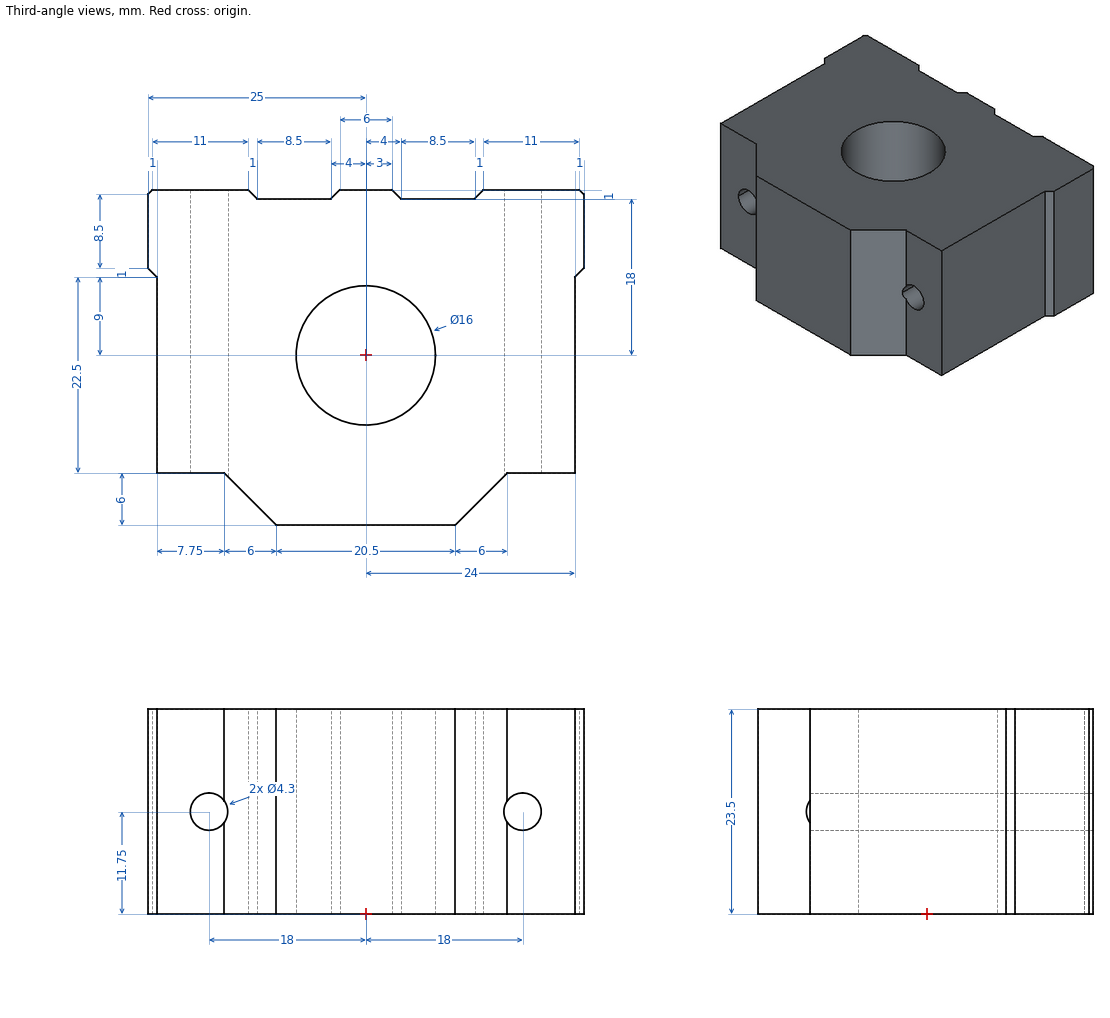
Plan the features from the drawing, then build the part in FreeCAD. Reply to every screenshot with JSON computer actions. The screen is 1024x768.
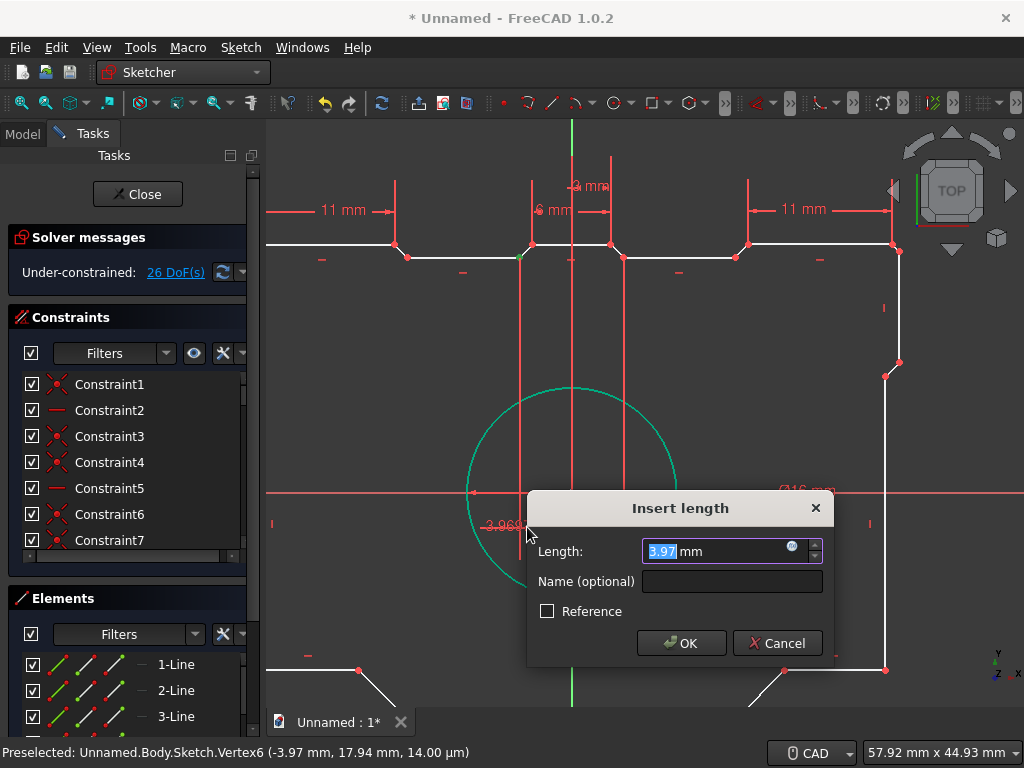
{"action": "type", "text": "4"}
{"action": "key", "text": "Return"}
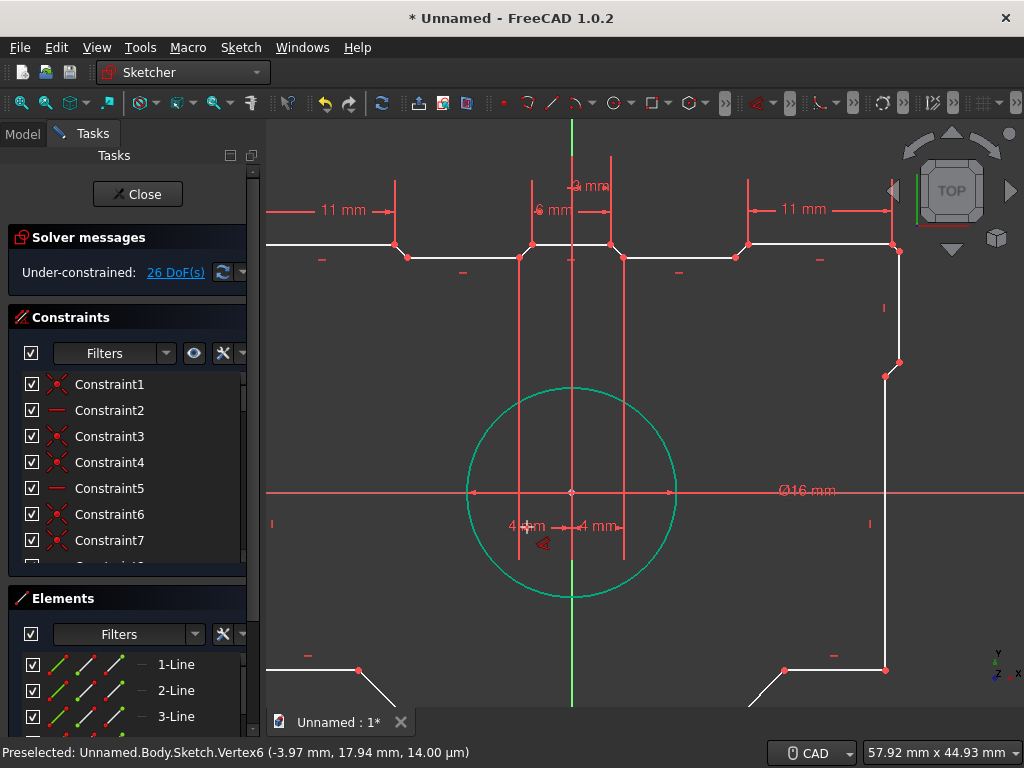
{"action": "scroll", "coordinate": [586, 244], "scroll_direction": "down", "scroll_amount": 2}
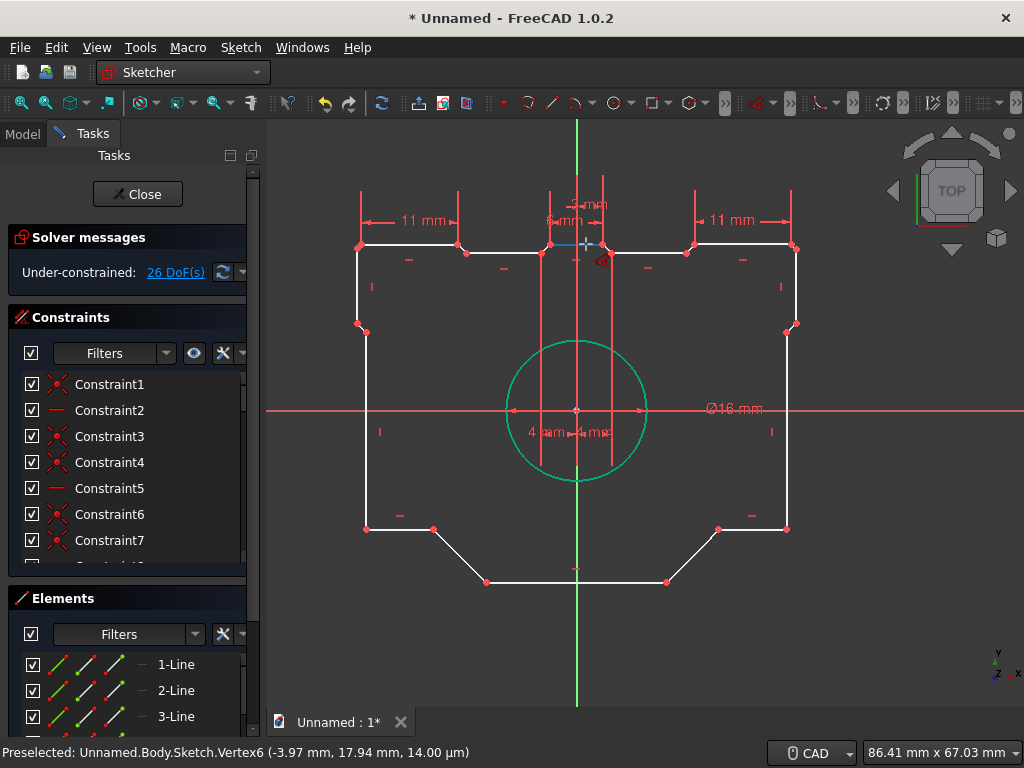
{"action": "left_click", "coordinate": [366, 332]}
{"action": "left_click", "coordinate": [332, 371]}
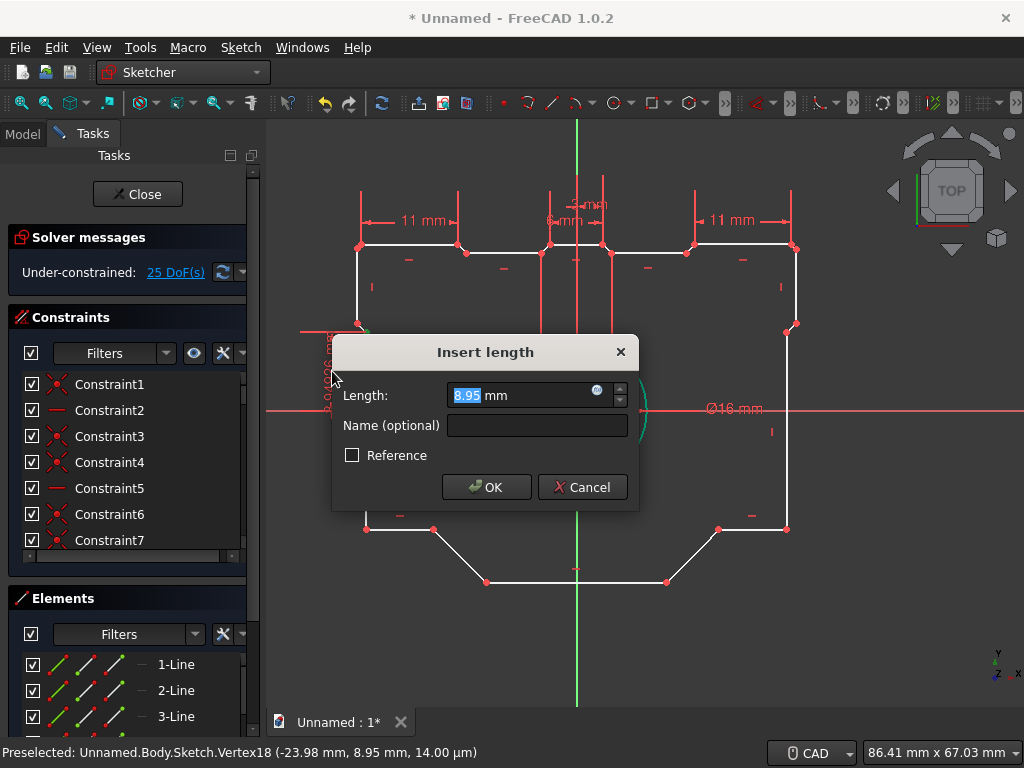
{"action": "type", "text": "9"}
{"action": "key", "text": "Return"}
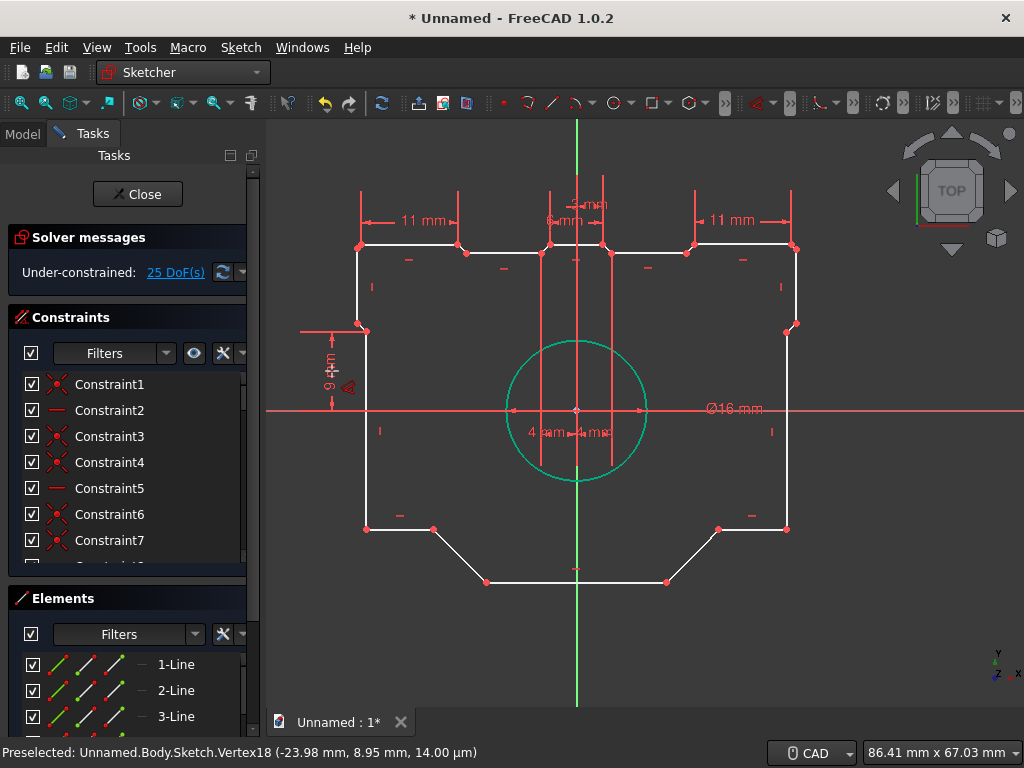
{"action": "left_click", "coordinate": [787, 333]}
{"action": "left_click", "coordinate": [821, 372]}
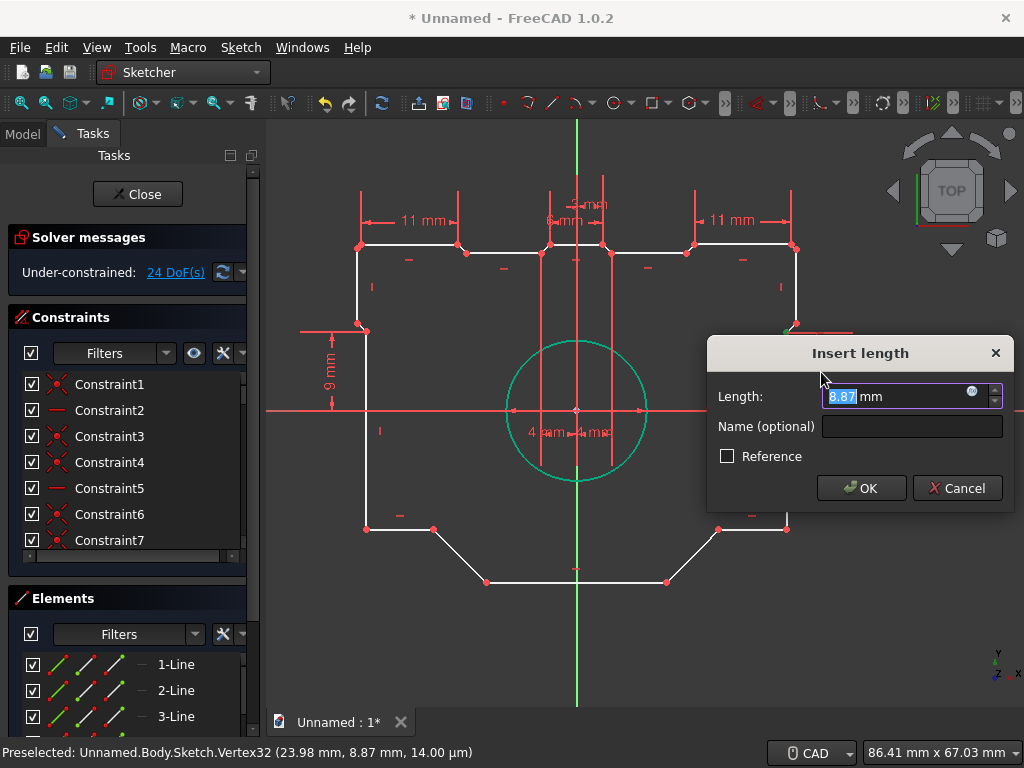
{"action": "type", "text": "9"}
{"action": "key", "text": "Return"}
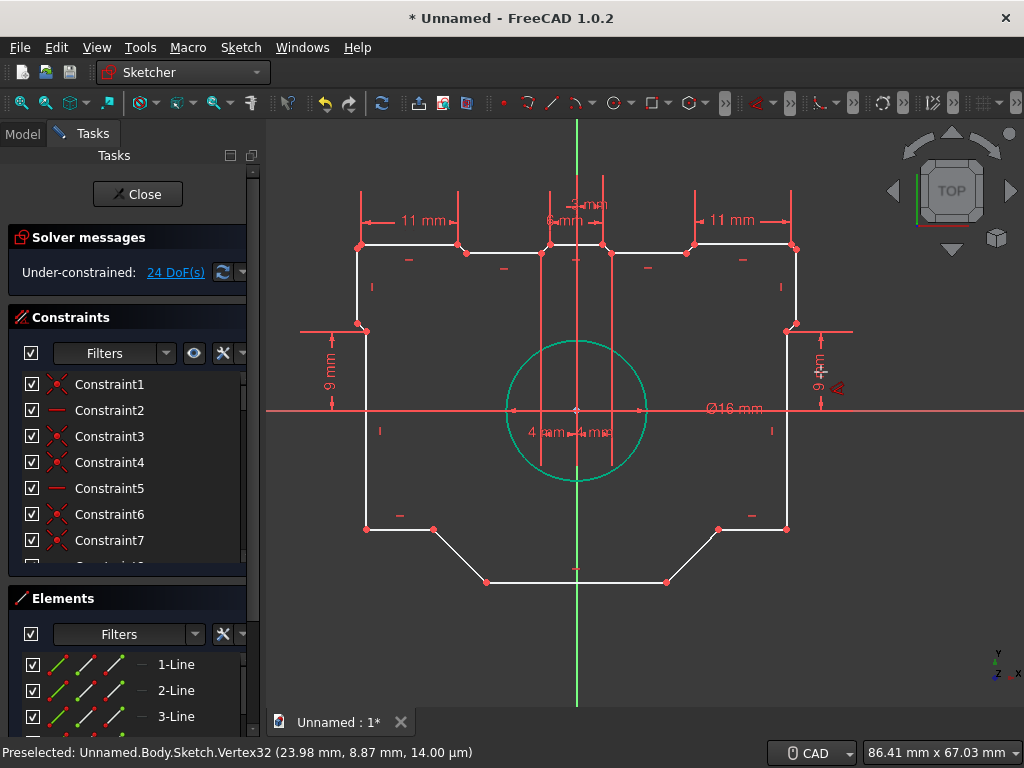
{"action": "scroll", "coordinate": [607, 249], "scroll_direction": "up", "scroll_amount": 8}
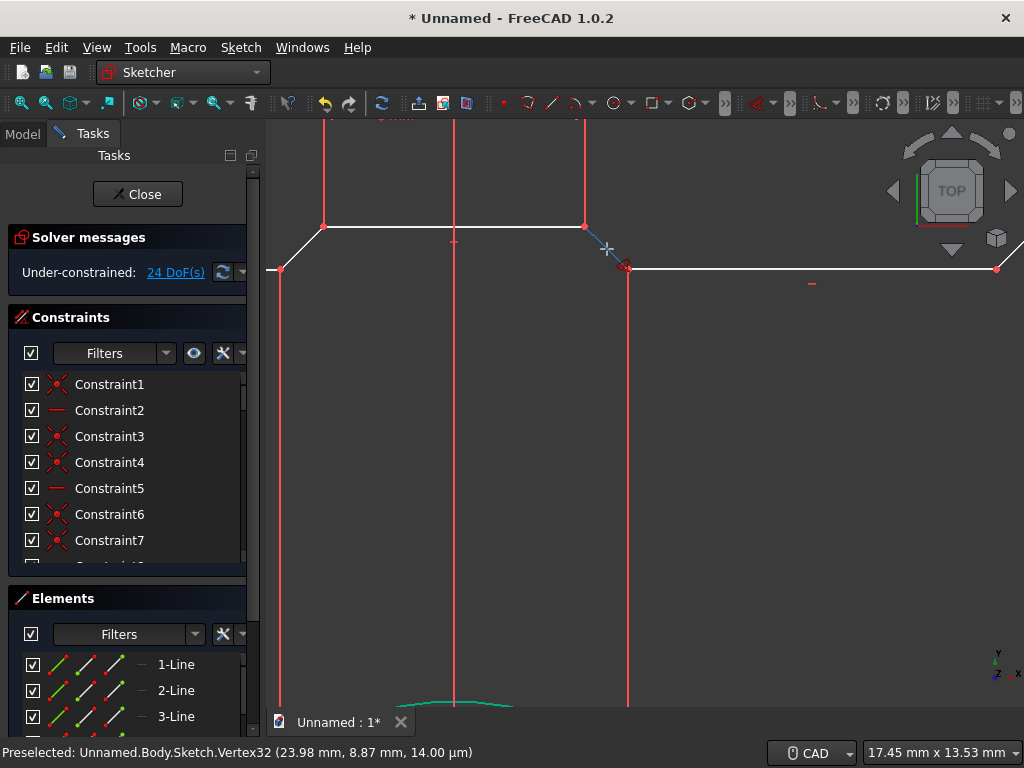
{"action": "left_click", "coordinate": [606, 248]}
{"action": "left_click", "coordinate": [662, 248]}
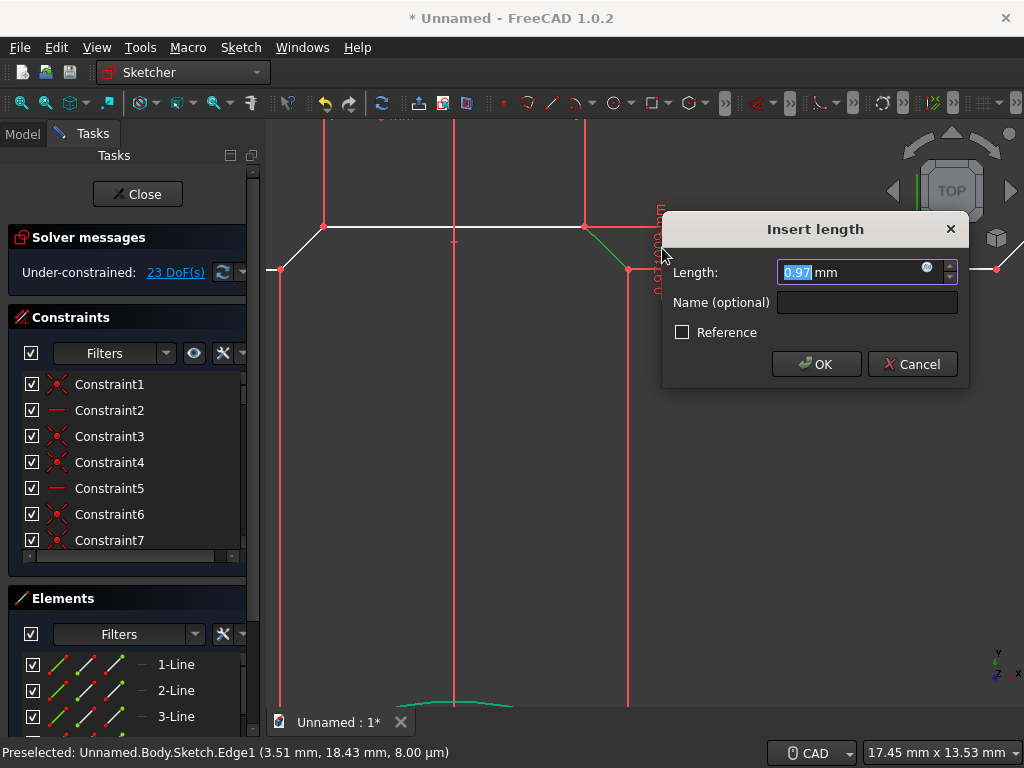
{"action": "type", "text": "1"}
{"action": "key", "text": "Return"}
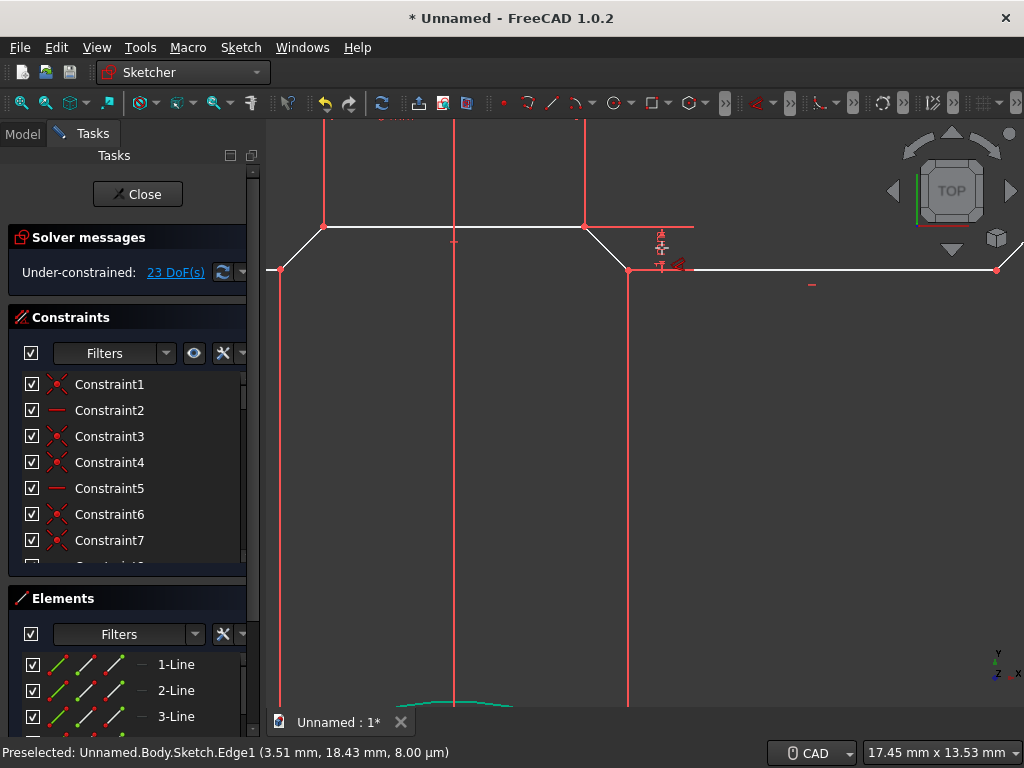
{"action": "left_click", "coordinate": [311, 240]}
{"action": "left_click", "coordinate": [358, 248]}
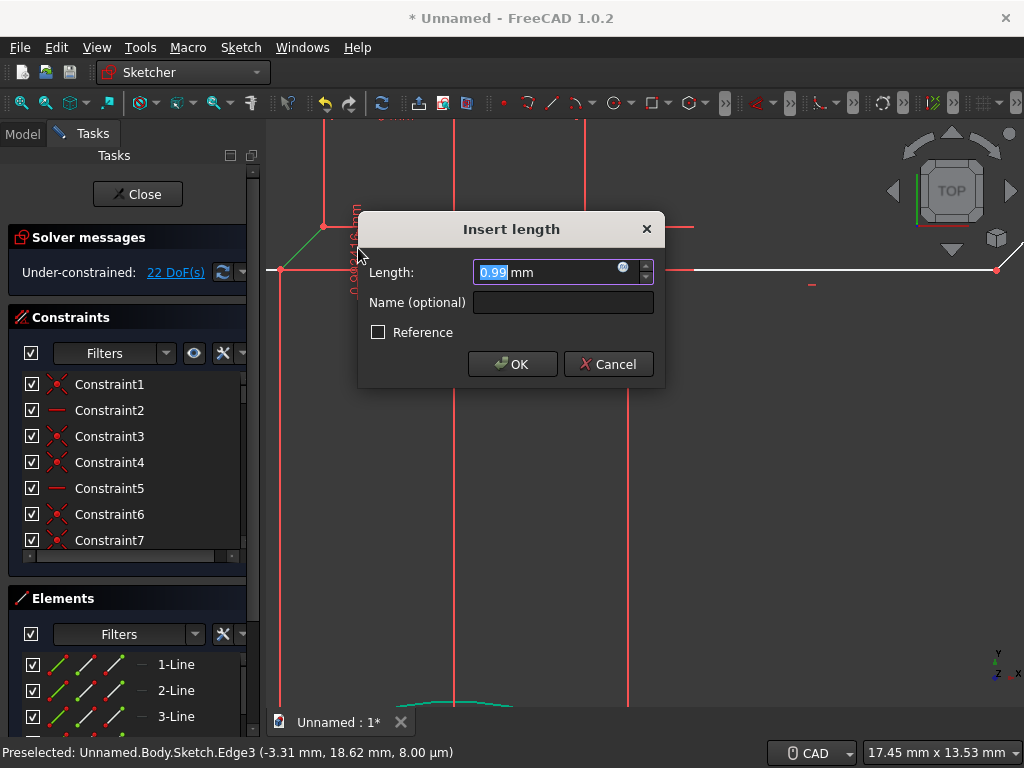
{"action": "type", "text": "1"}
{"action": "key", "text": "Return"}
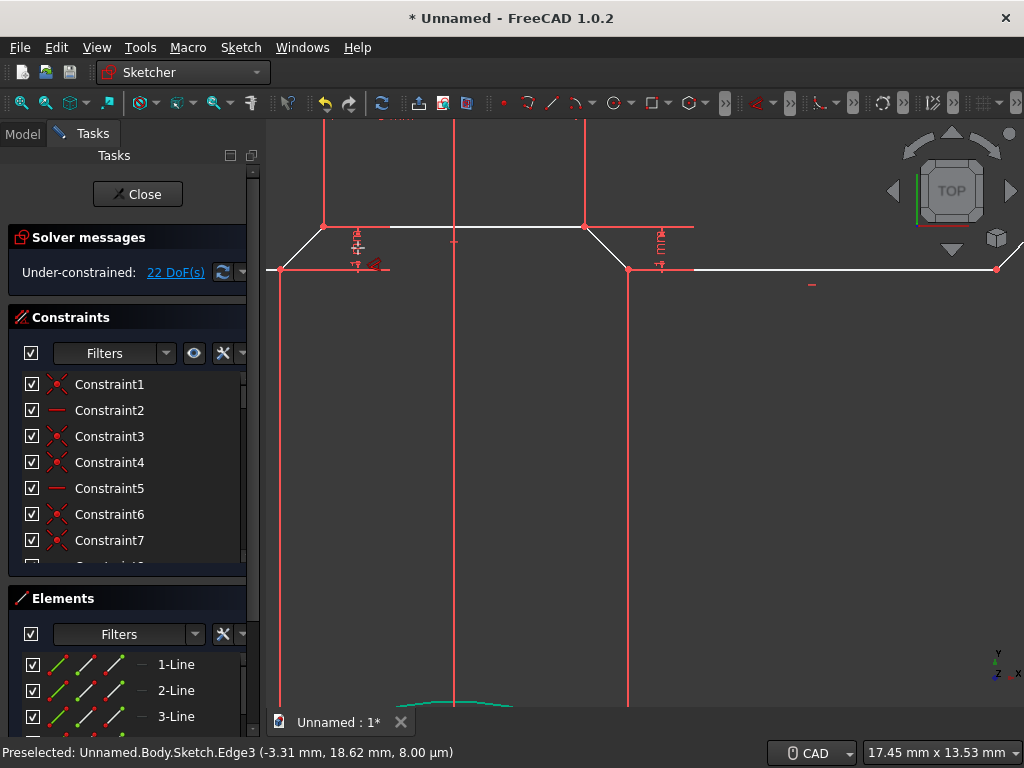
{"action": "scroll", "coordinate": [607, 249], "scroll_direction": "down", "scroll_amount": 8}